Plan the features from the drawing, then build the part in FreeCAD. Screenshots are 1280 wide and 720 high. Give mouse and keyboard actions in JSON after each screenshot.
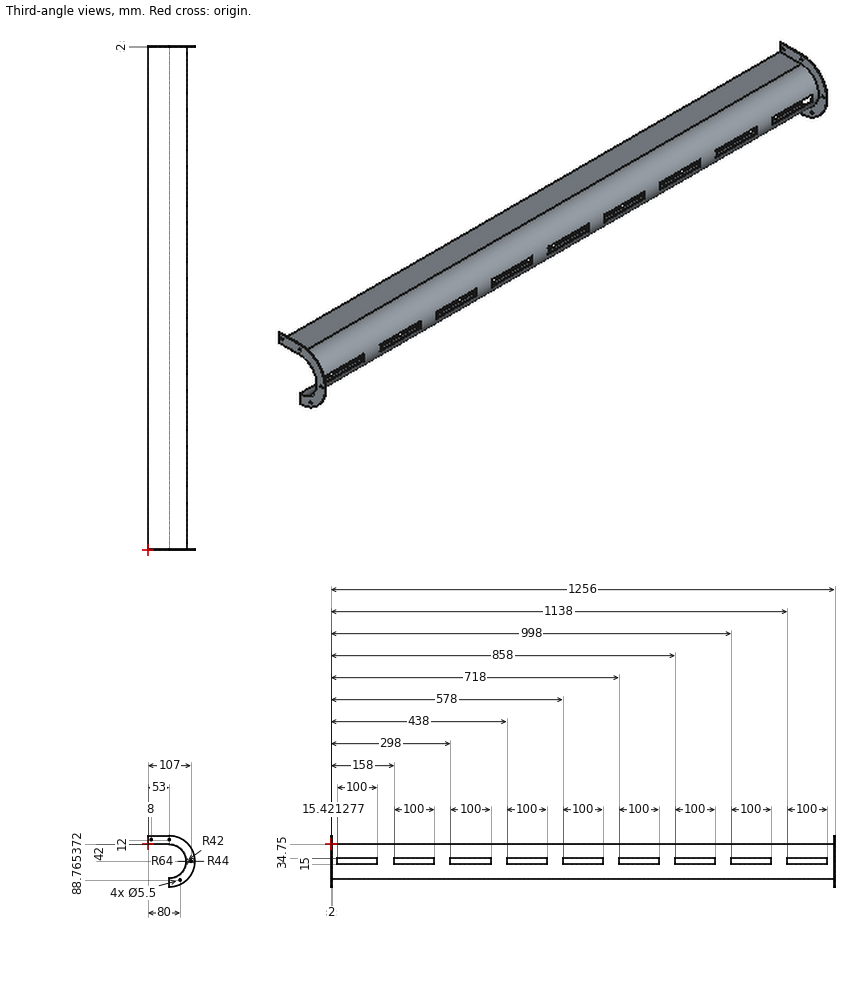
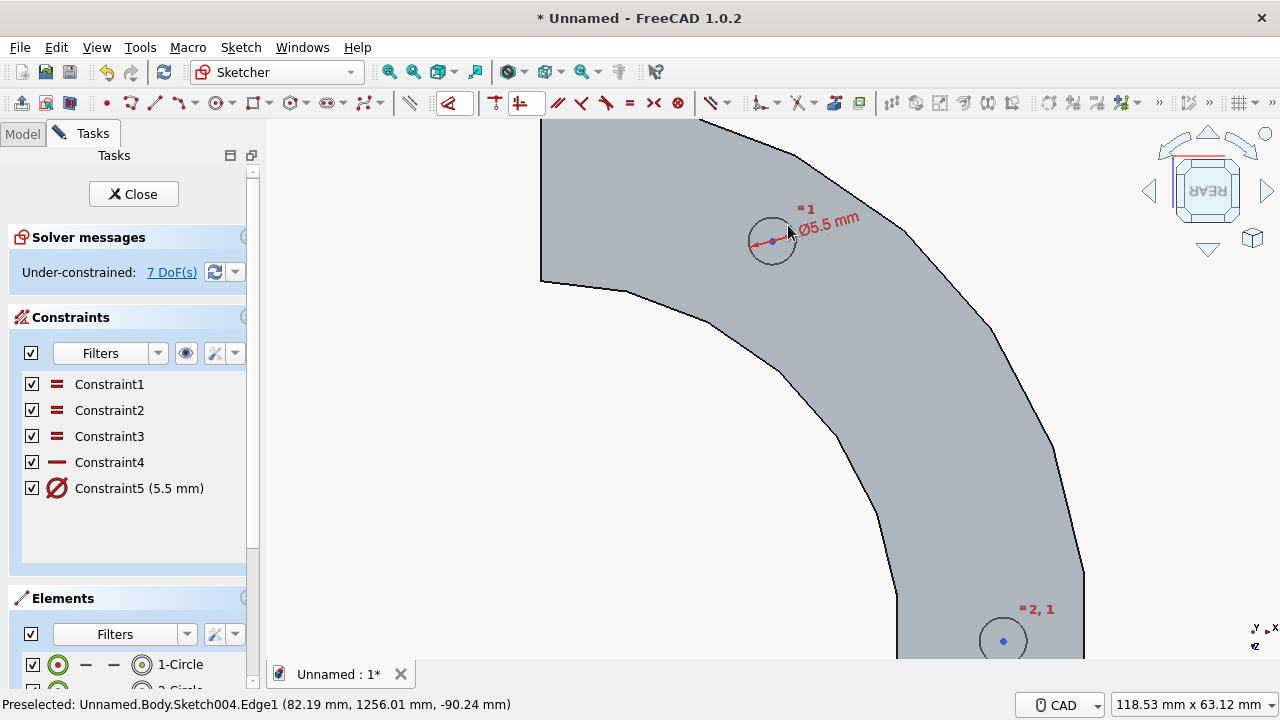
{"action": "scroll", "coordinate": [790, 225], "scroll_direction": "down", "scroll_amount": 5}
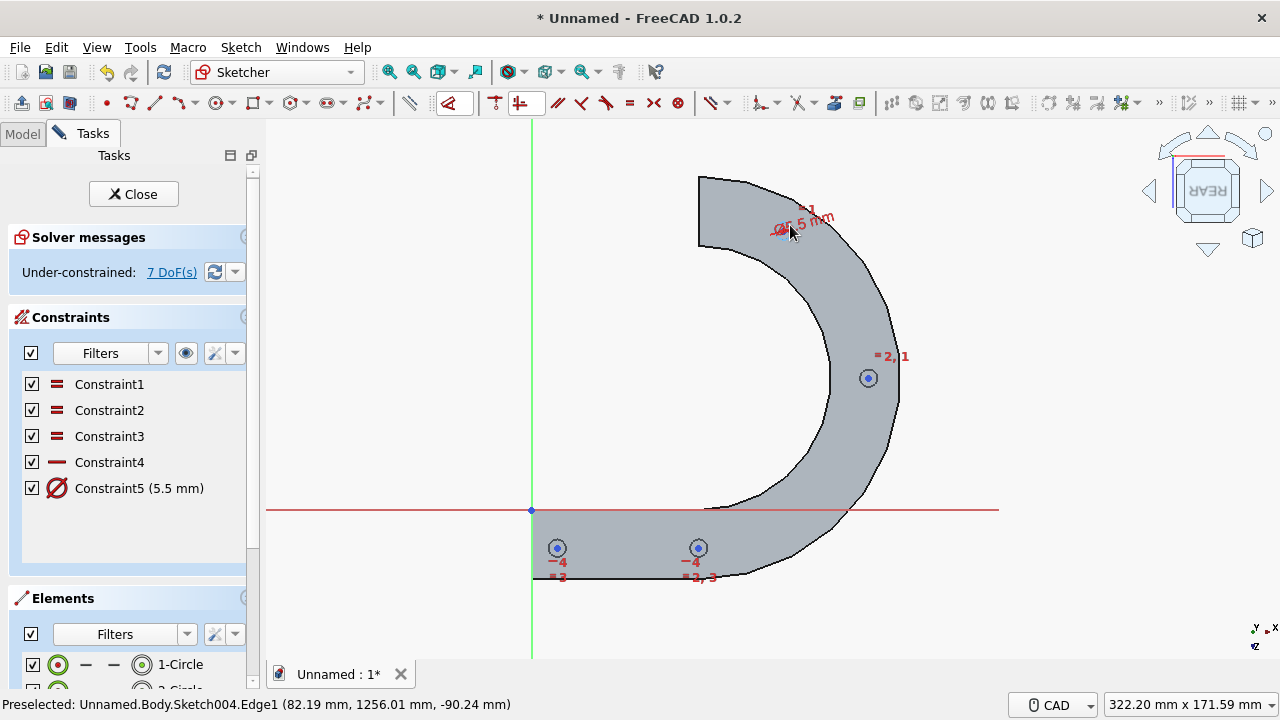
{"action": "scroll", "coordinate": [557, 548], "scroll_direction": "up", "scroll_amount": 3}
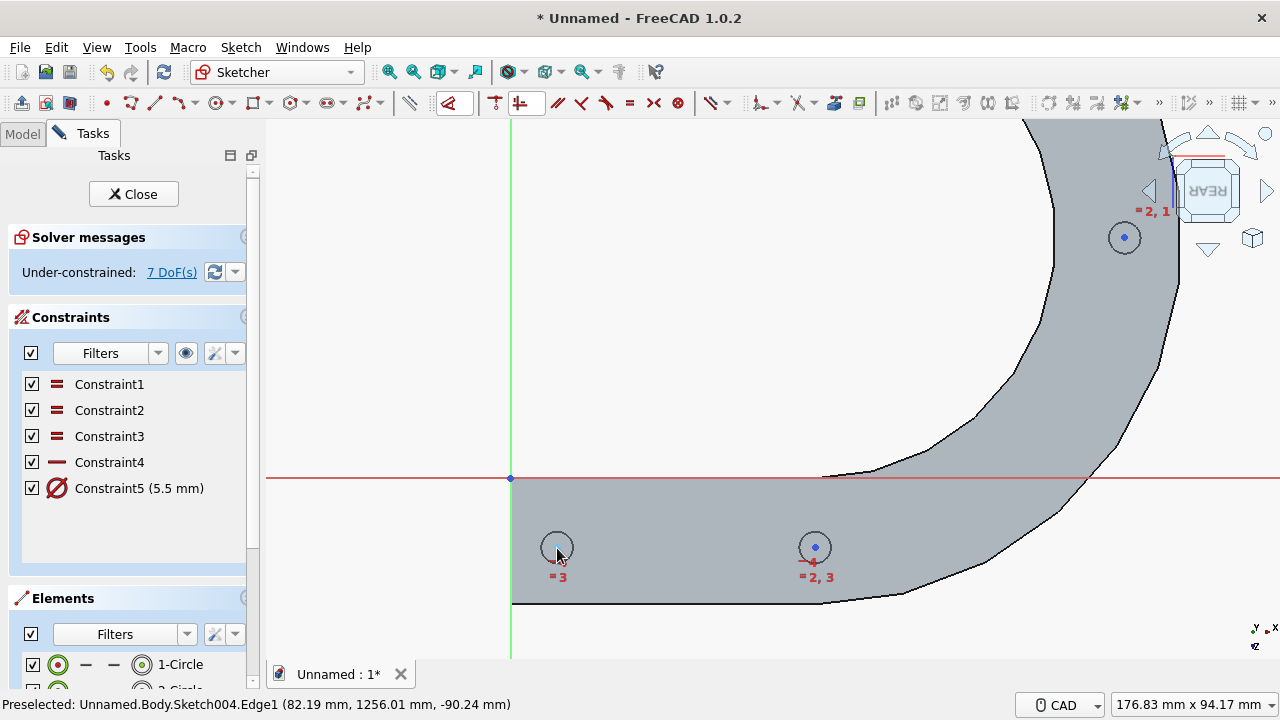
{"action": "left_click", "coordinate": [557, 548]}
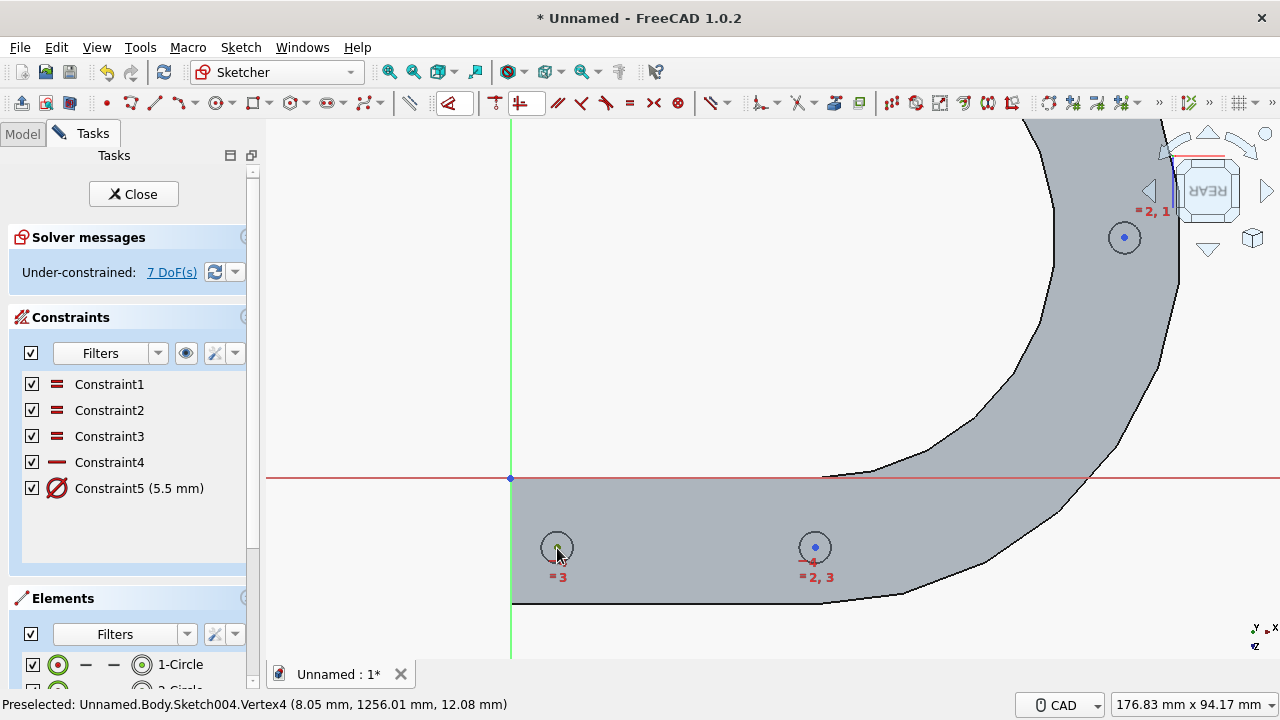
{"action": "key", "text": "l"}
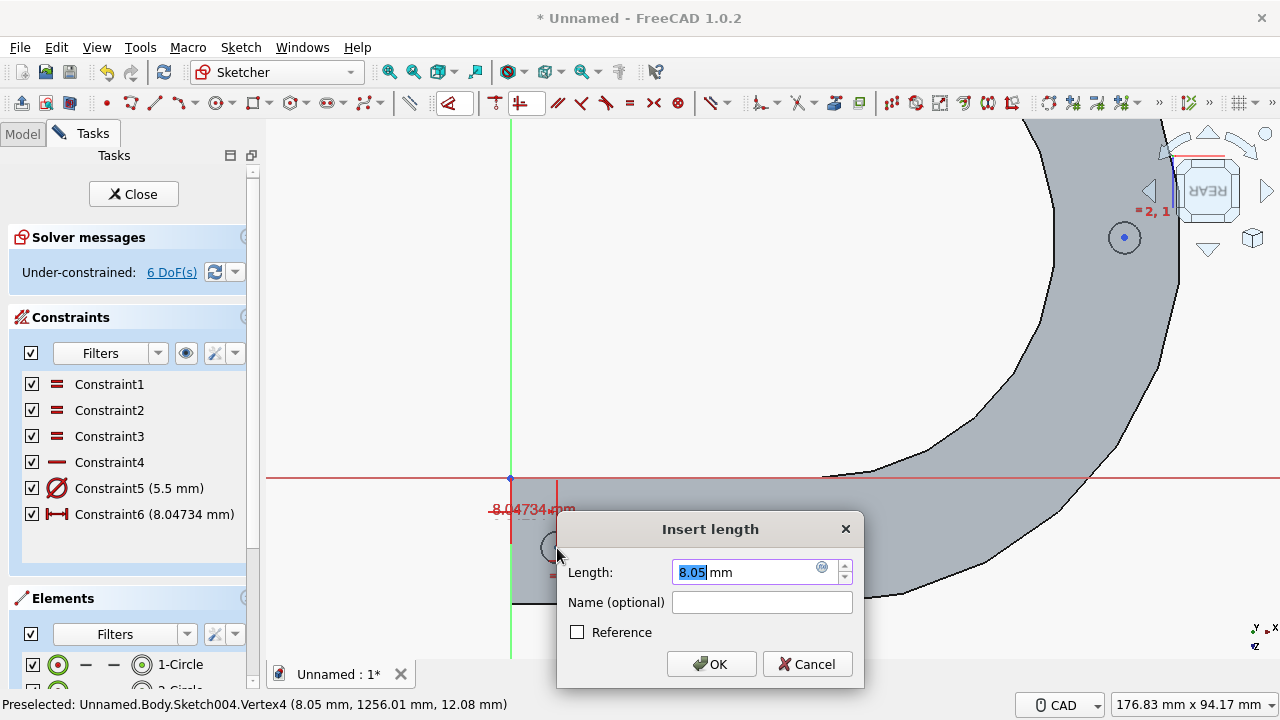
{"action": "type", "text": "8"}
{"action": "key", "text": "Return"}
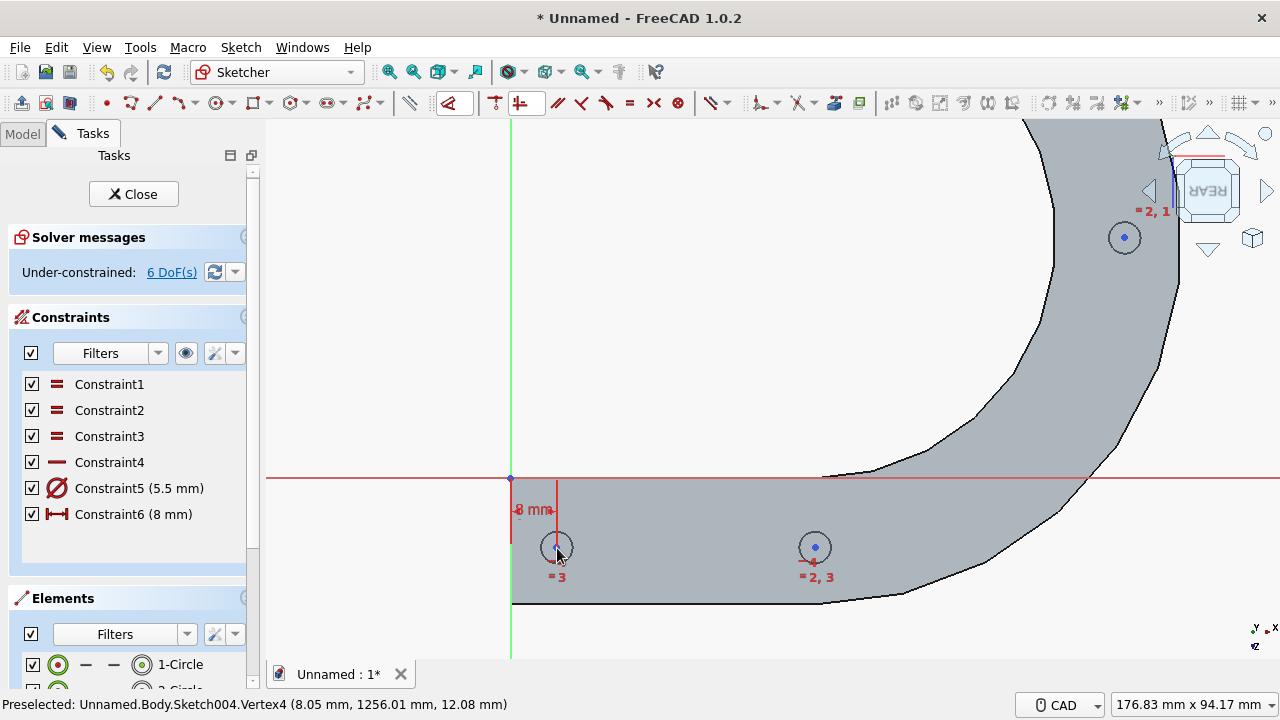
{"action": "scroll", "coordinate": [557, 548], "scroll_direction": "down", "scroll_amount": 3}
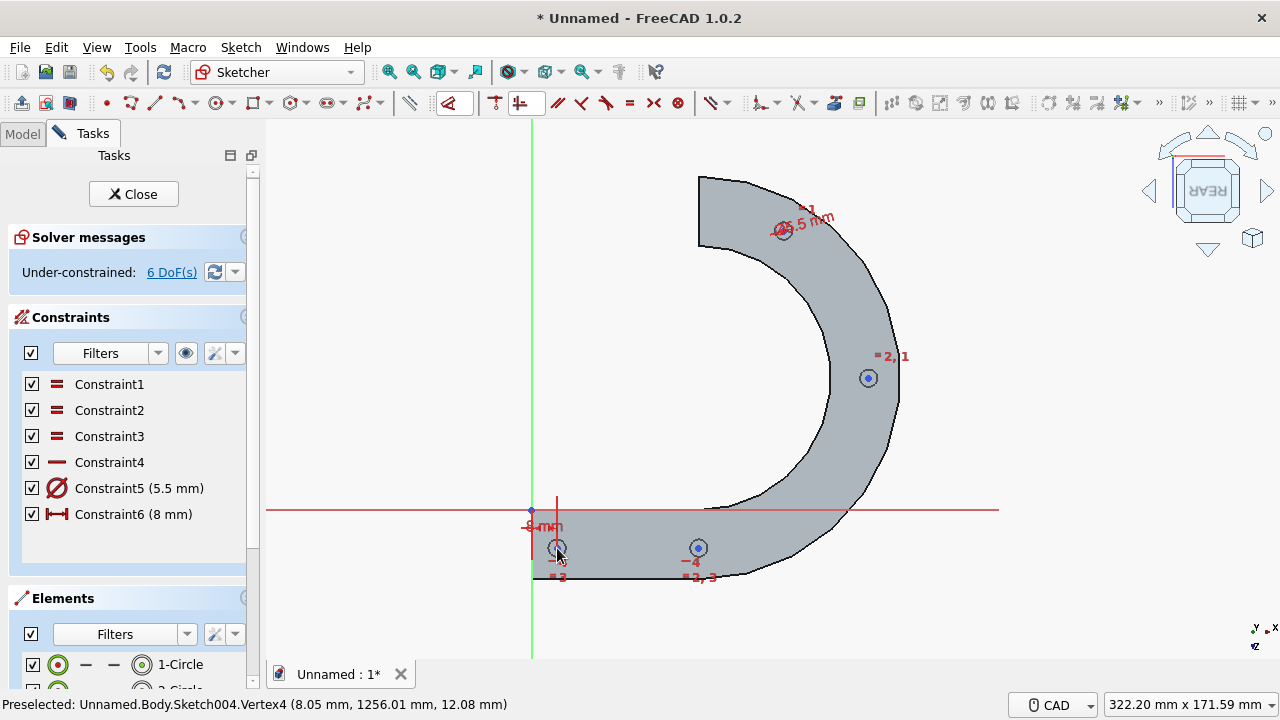
{"action": "left_click", "coordinate": [784, 231]}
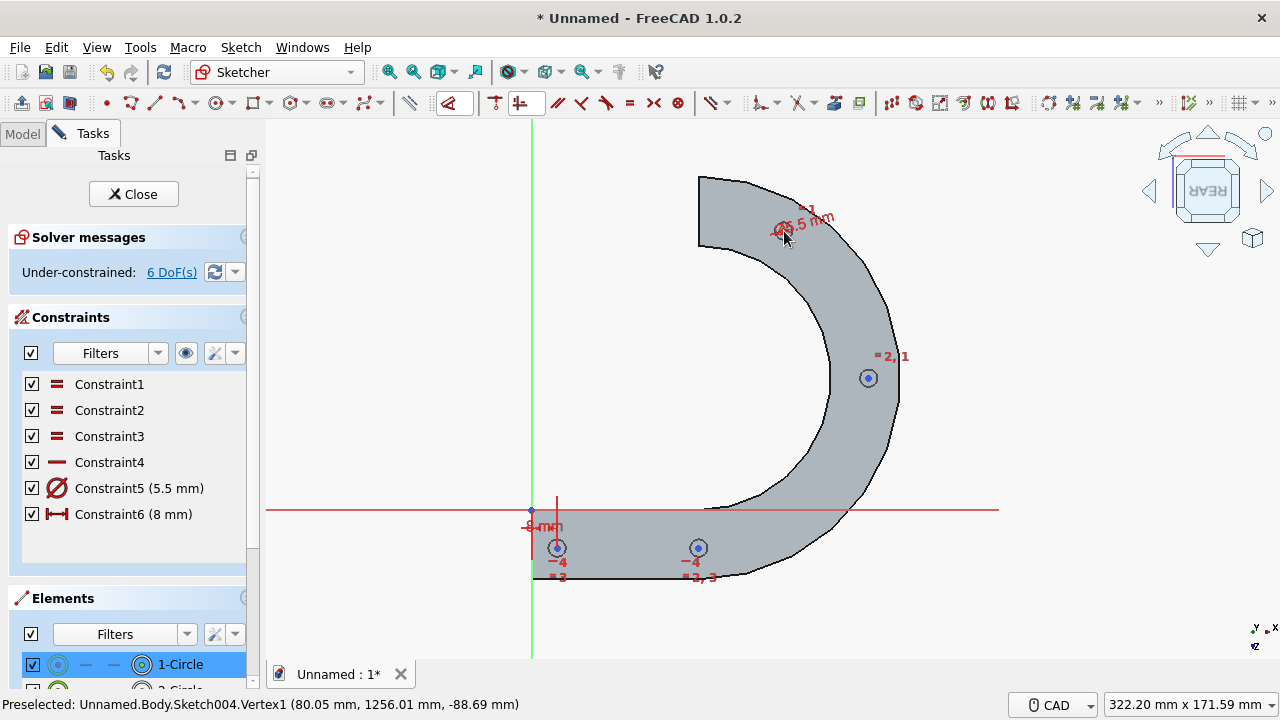
{"action": "left_click", "coordinate": [468, 104]}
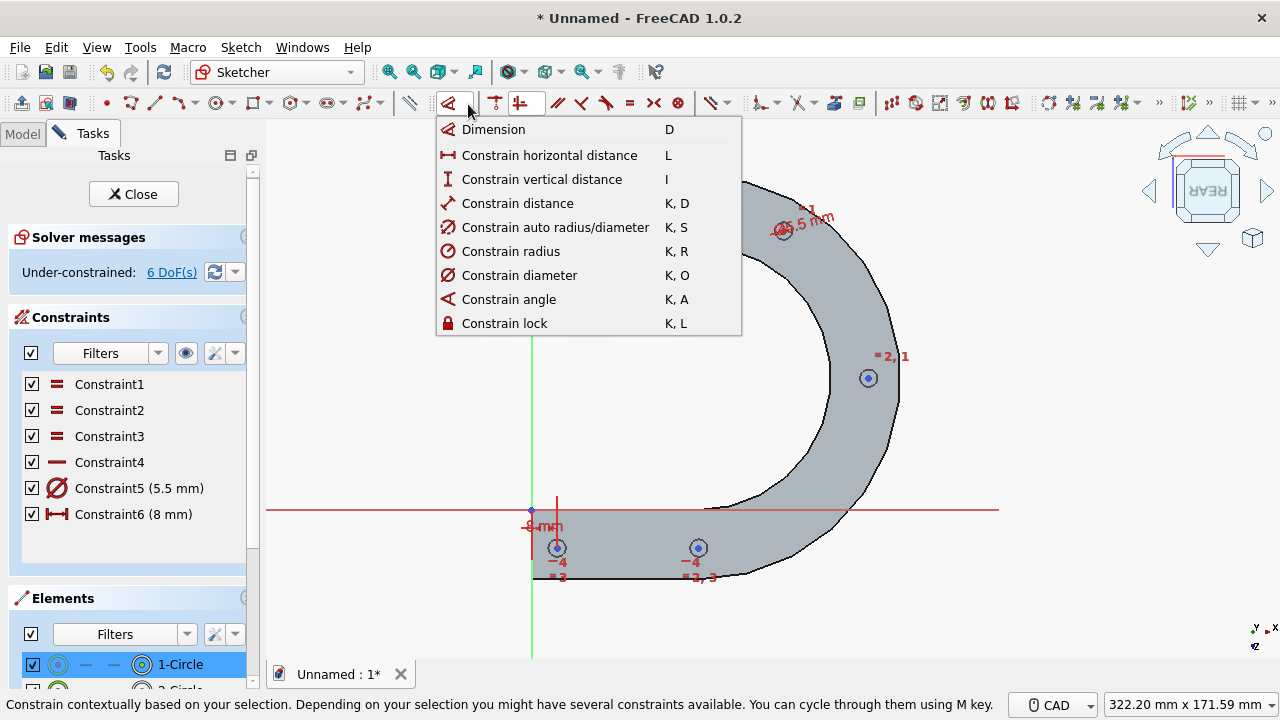
{"action": "left_click", "coordinate": [589, 155]}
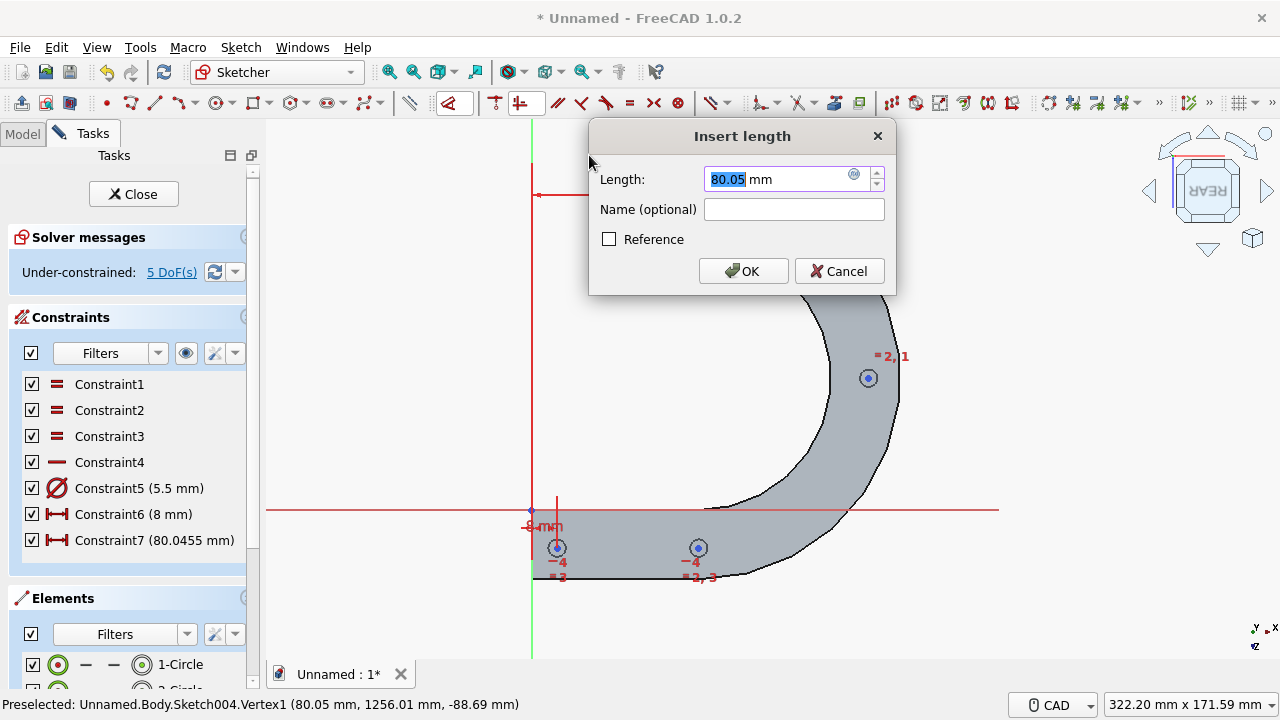
{"action": "type", "text": "80"}
{"action": "key", "text": "Return"}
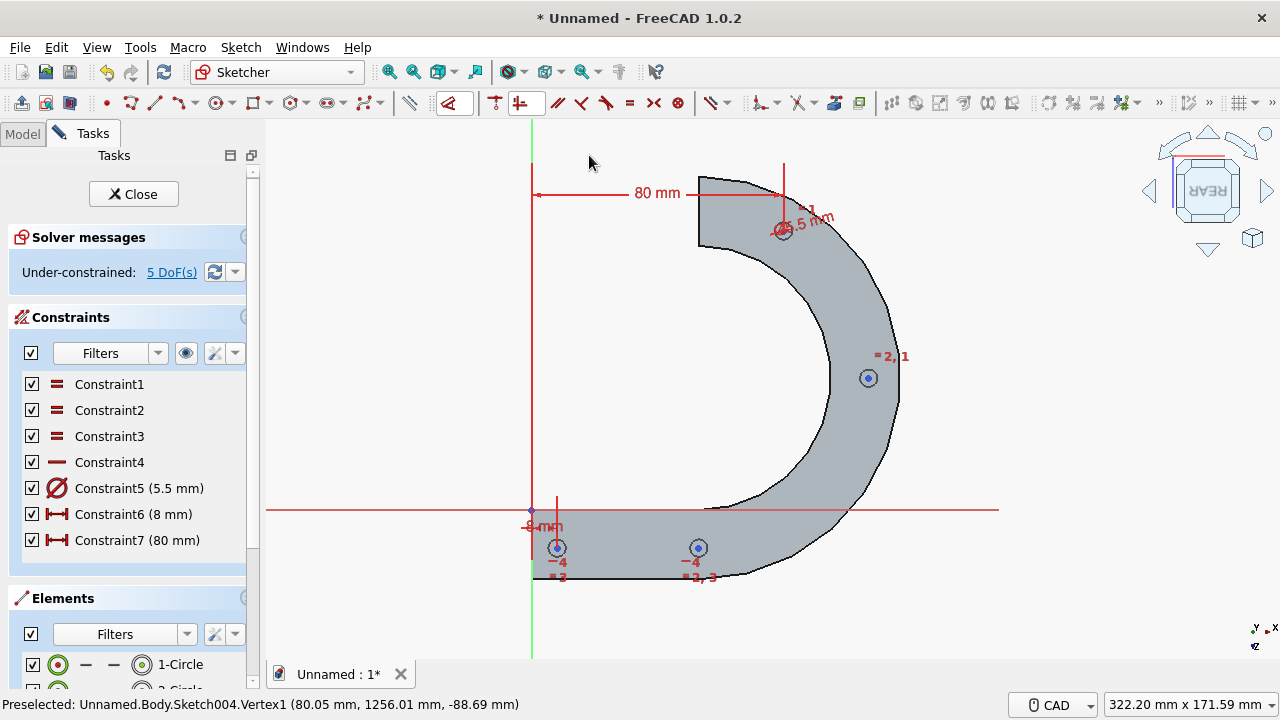
{"action": "left_click", "coordinate": [869, 378]}